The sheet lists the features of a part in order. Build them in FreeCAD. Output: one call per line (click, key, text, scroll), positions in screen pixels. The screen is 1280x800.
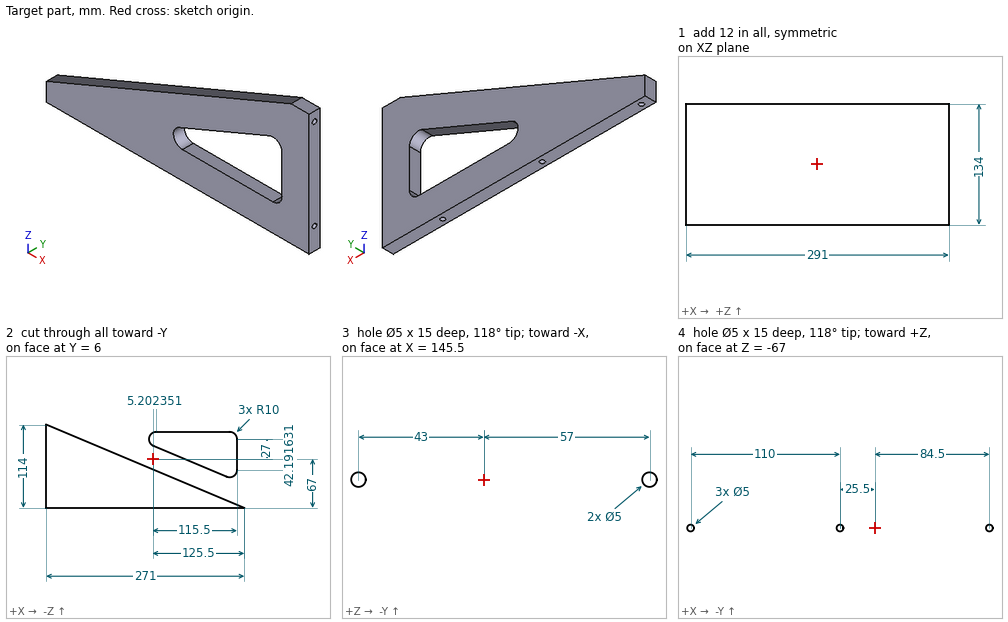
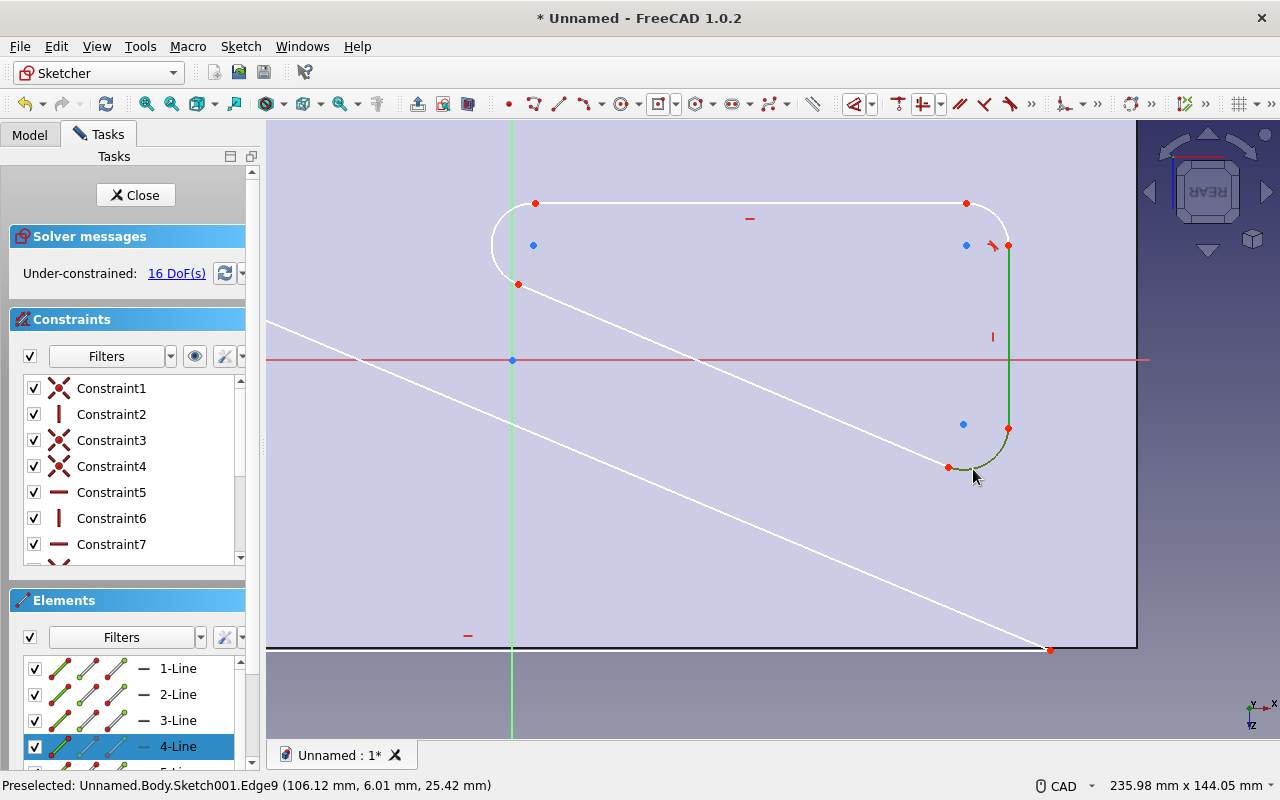
click(1010, 104)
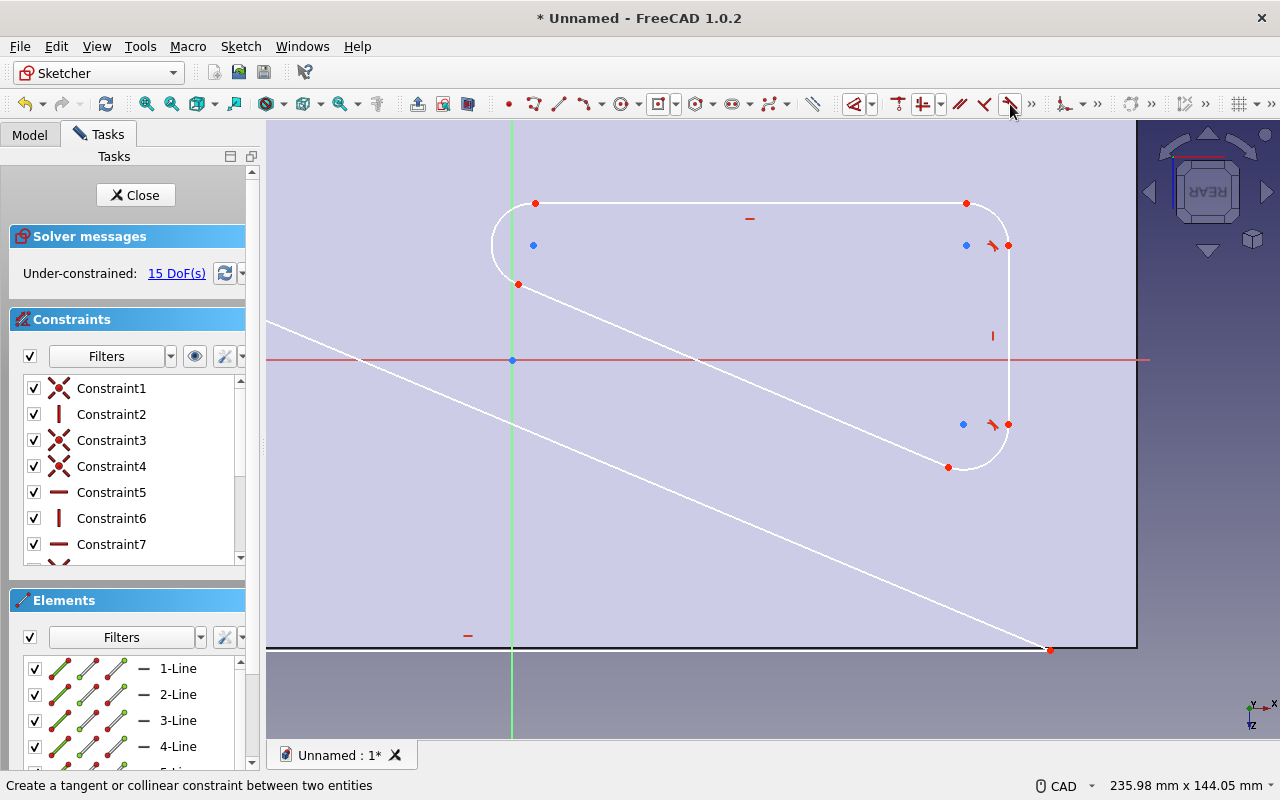
click(837, 203)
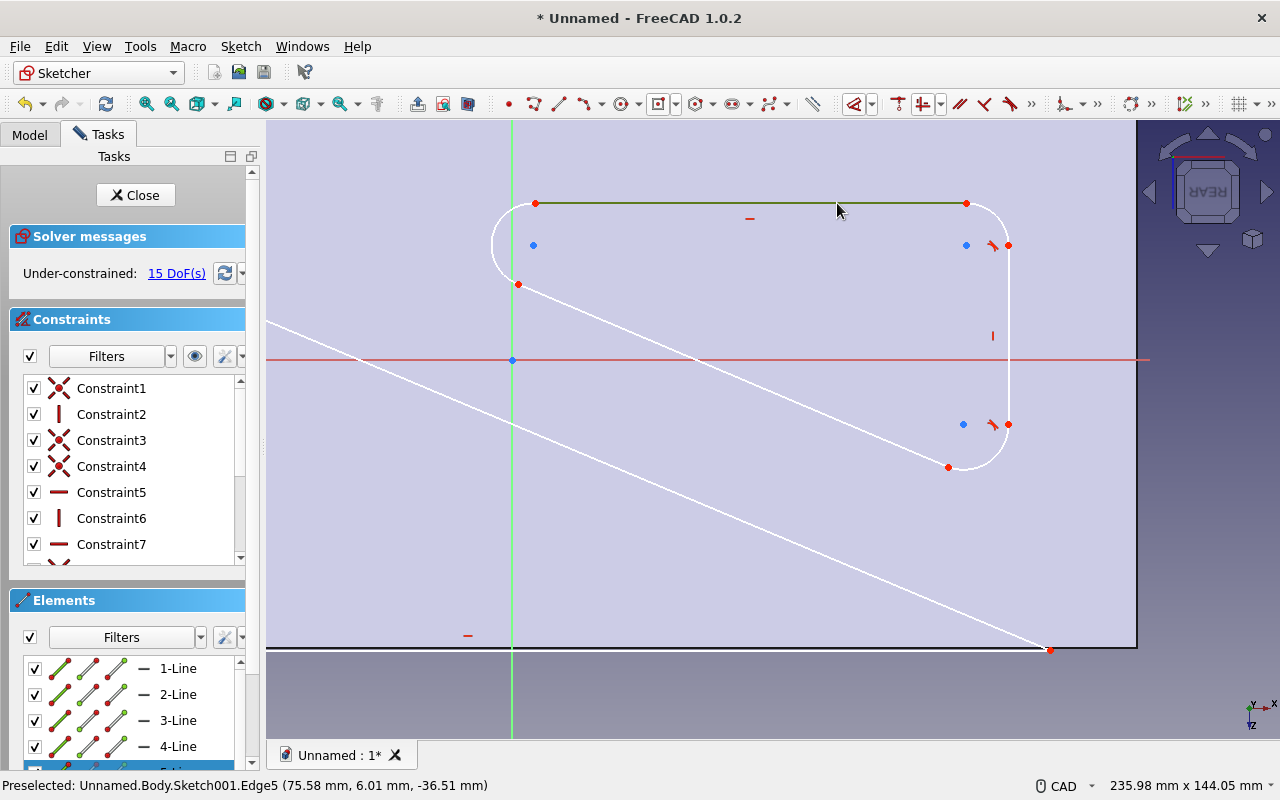
click(1004, 227)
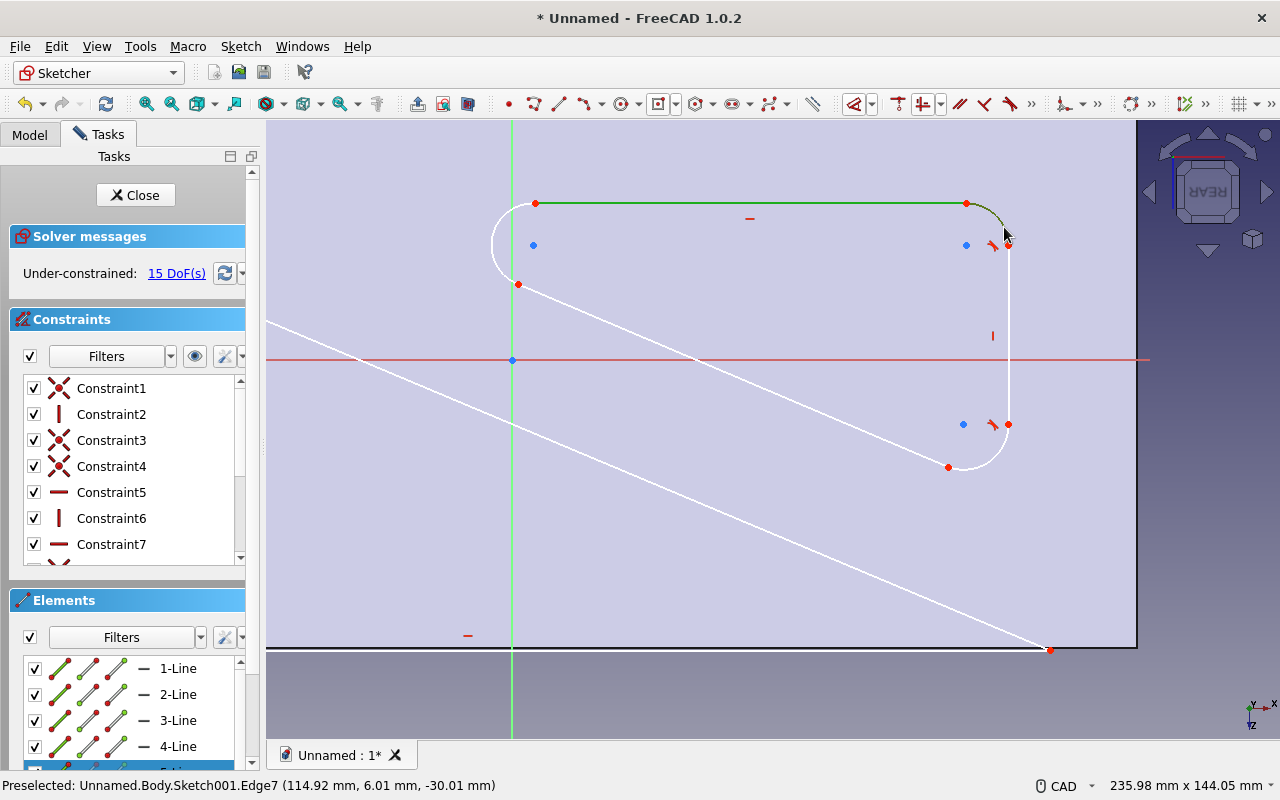
click(1010, 104)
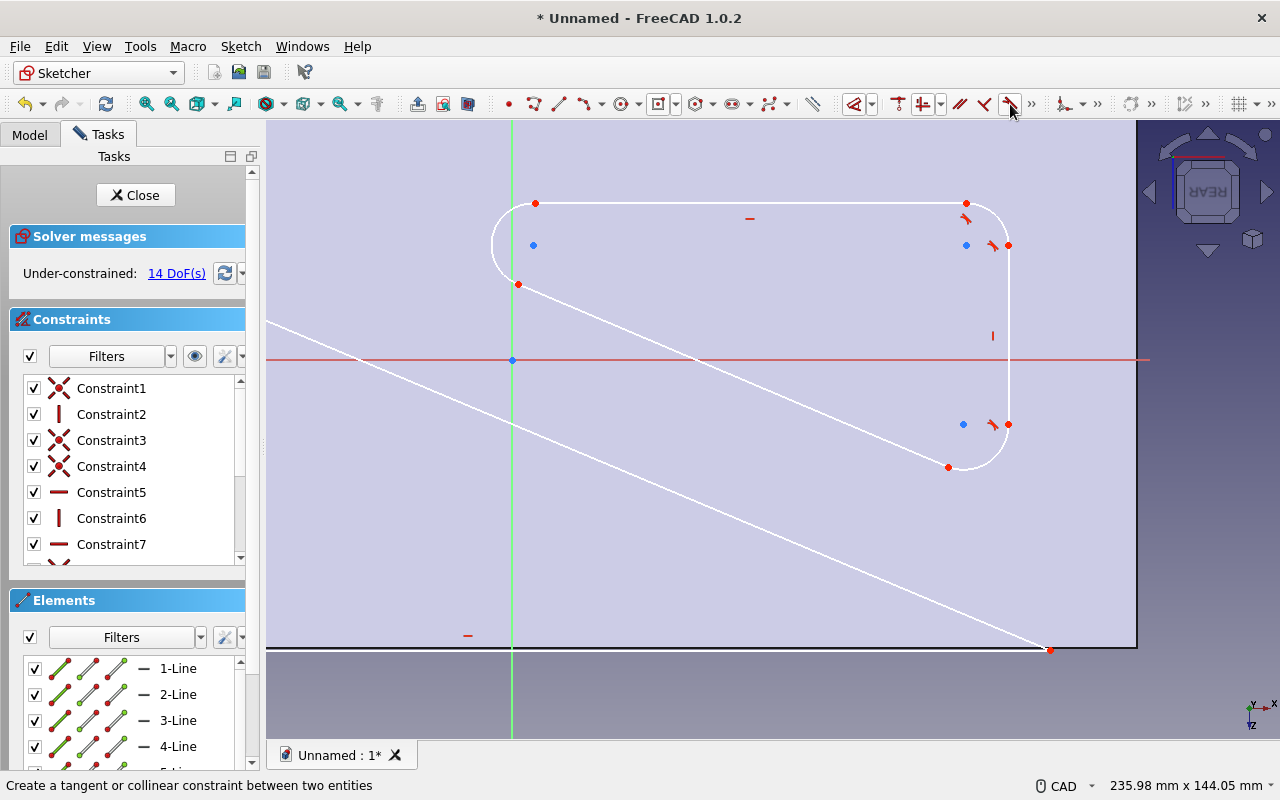
click(837, 203)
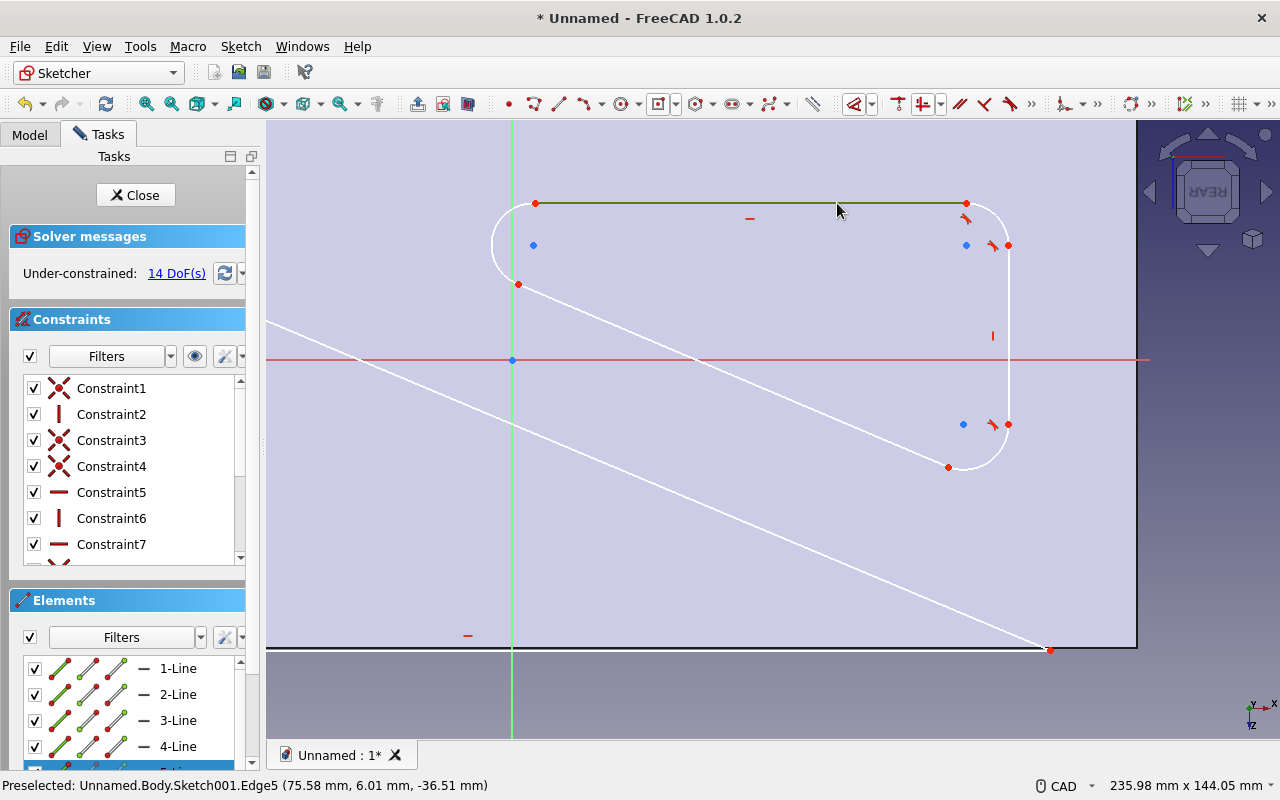
click(494, 260)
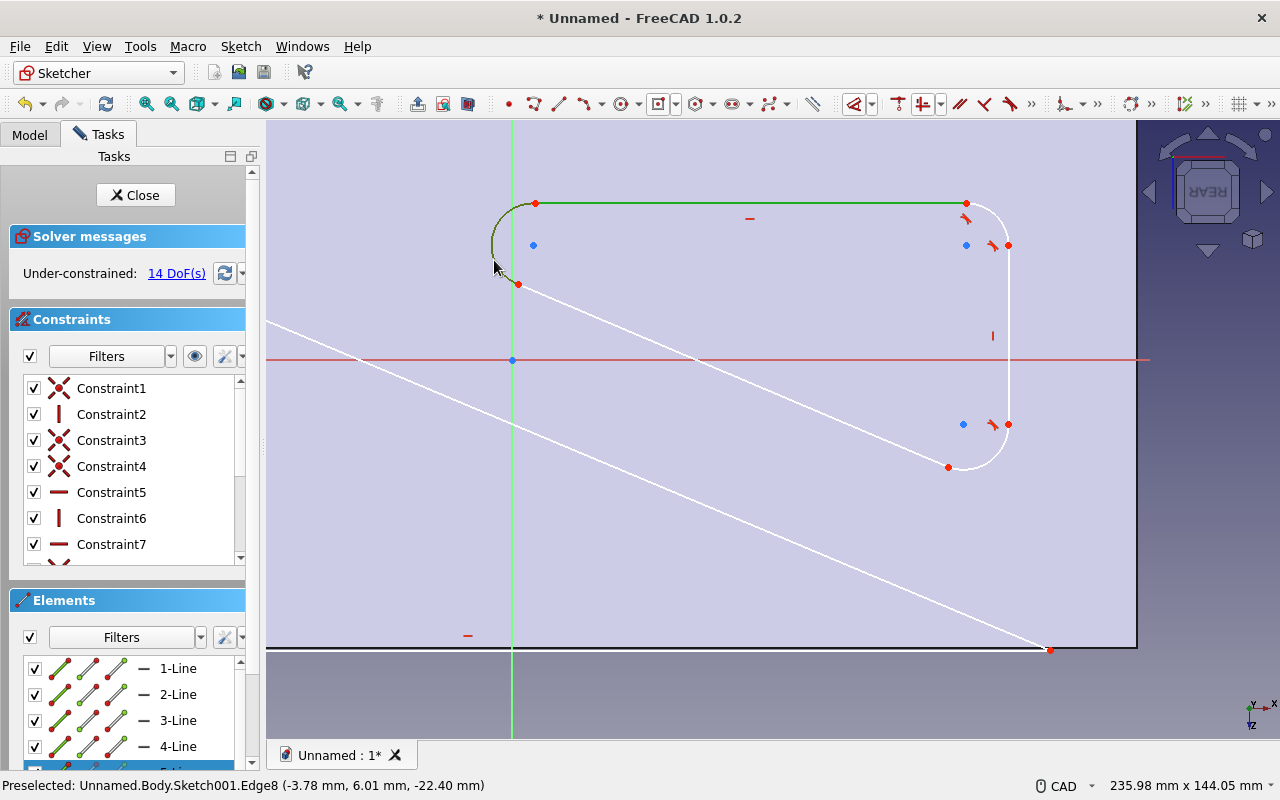
click(1010, 104)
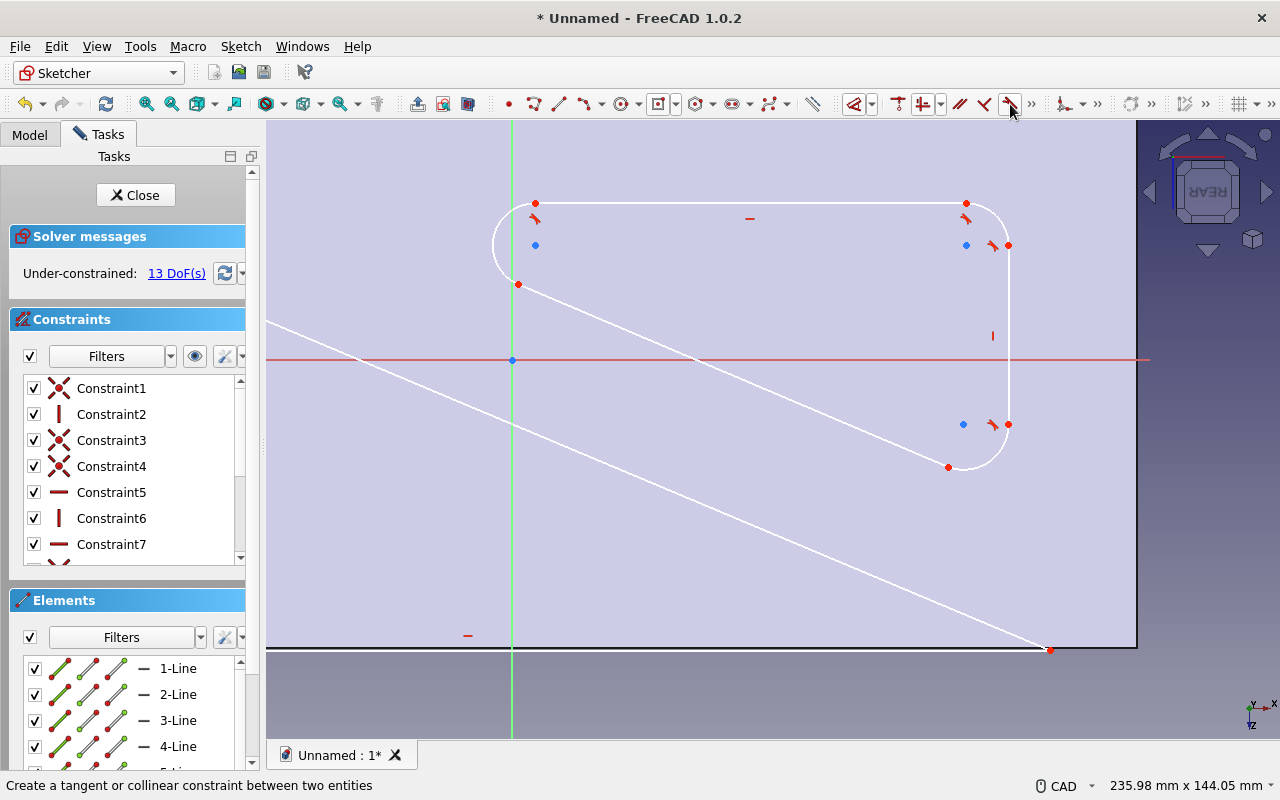
click(647, 339)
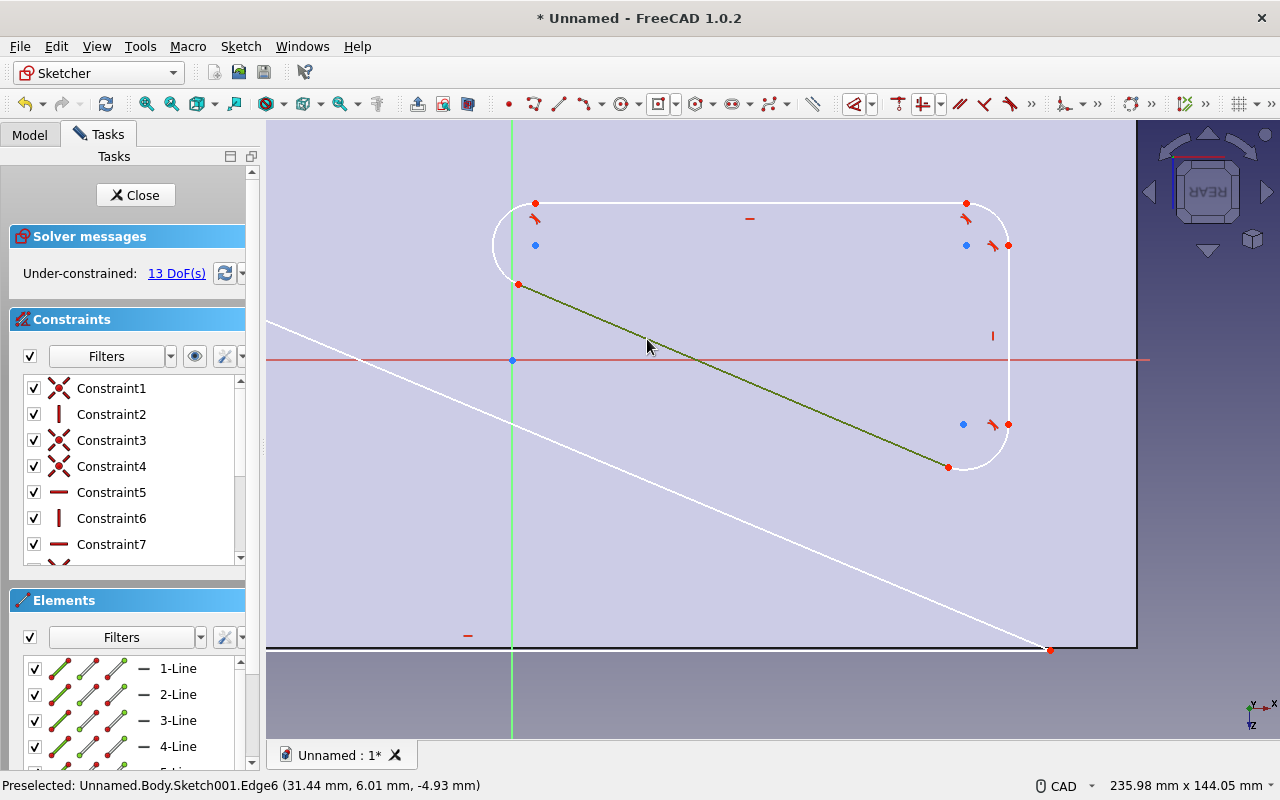
click(495, 260)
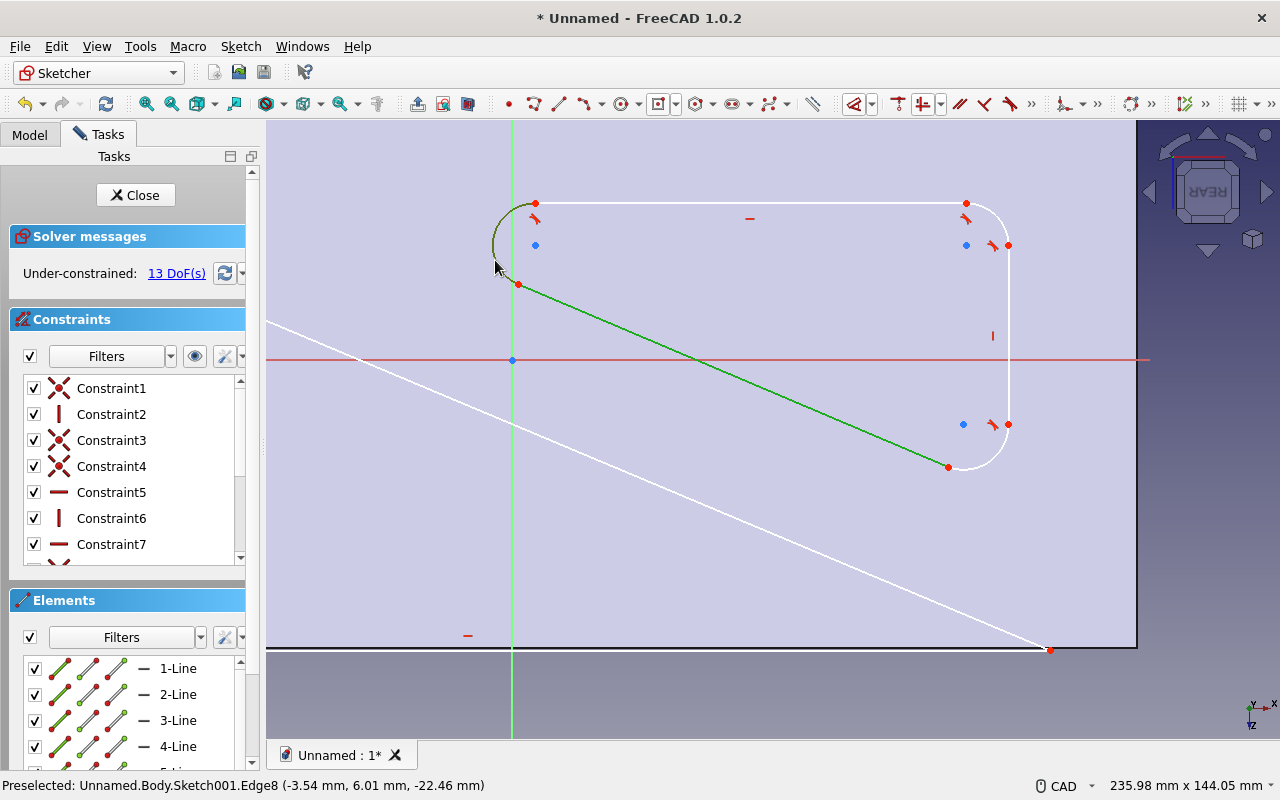
key(t)